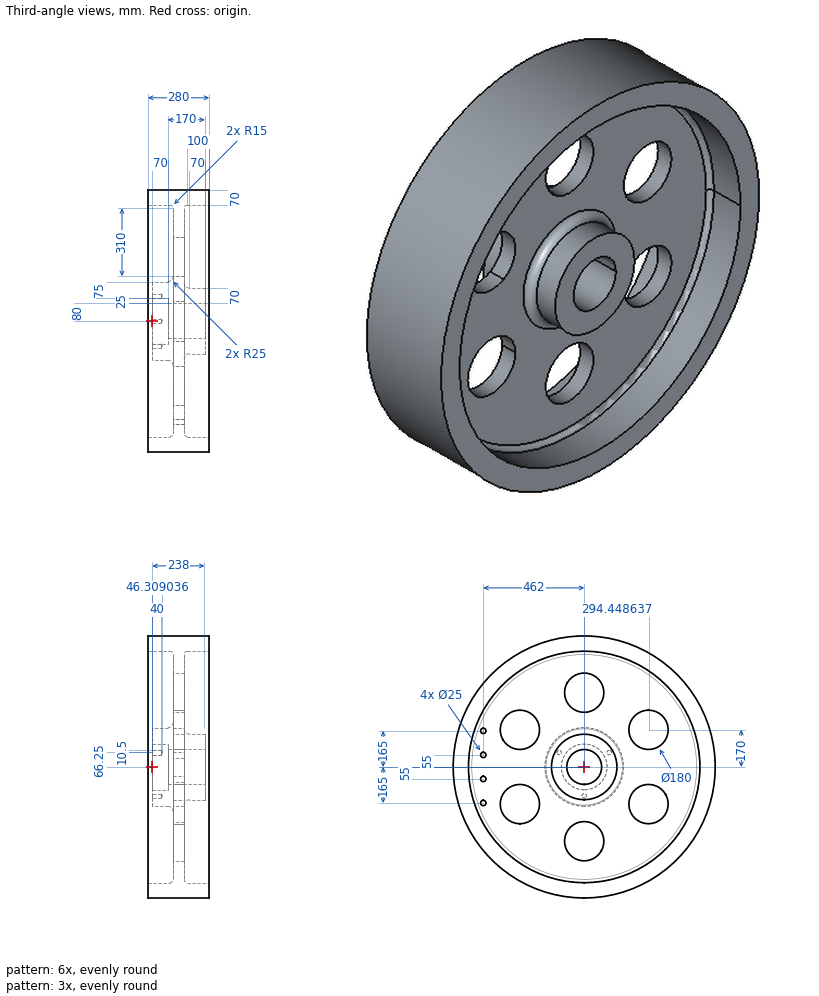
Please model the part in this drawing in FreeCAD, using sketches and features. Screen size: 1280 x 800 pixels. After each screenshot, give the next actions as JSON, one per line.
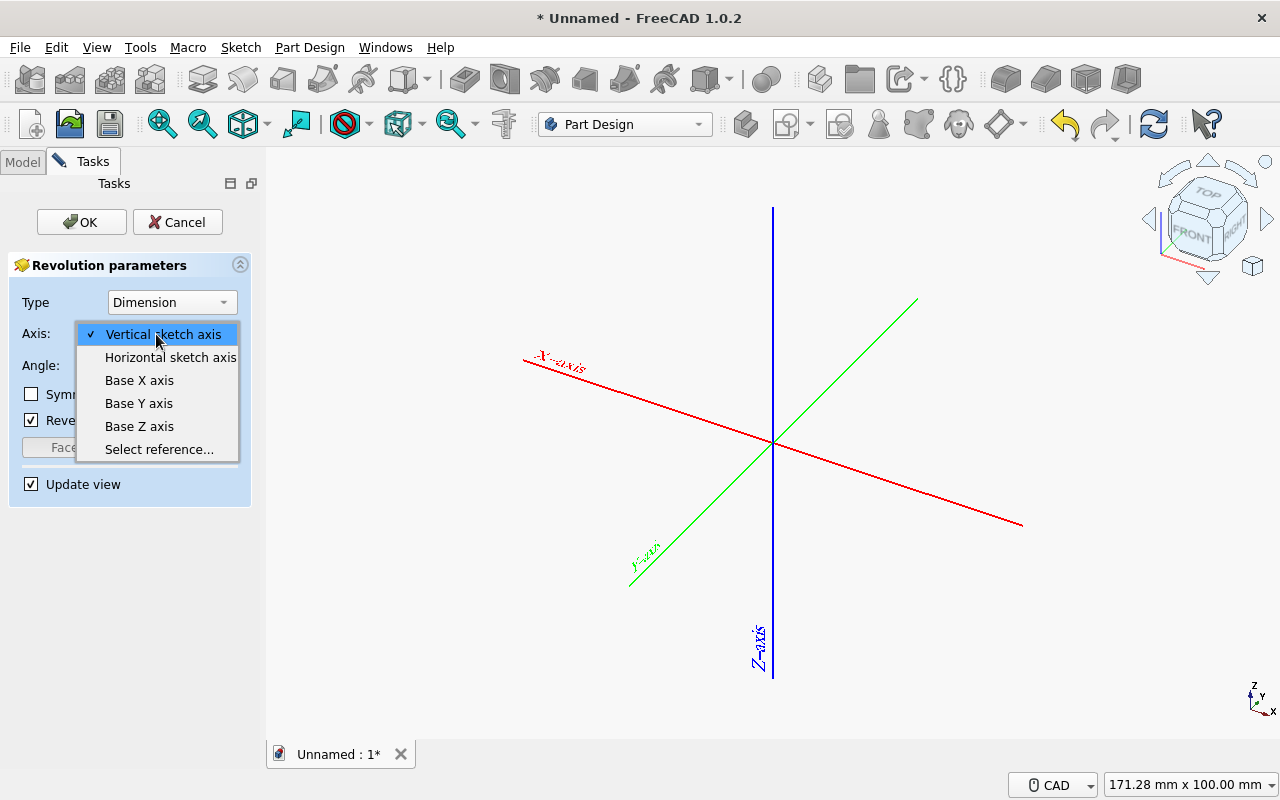
{"action": "left_click", "coordinate": [156, 358]}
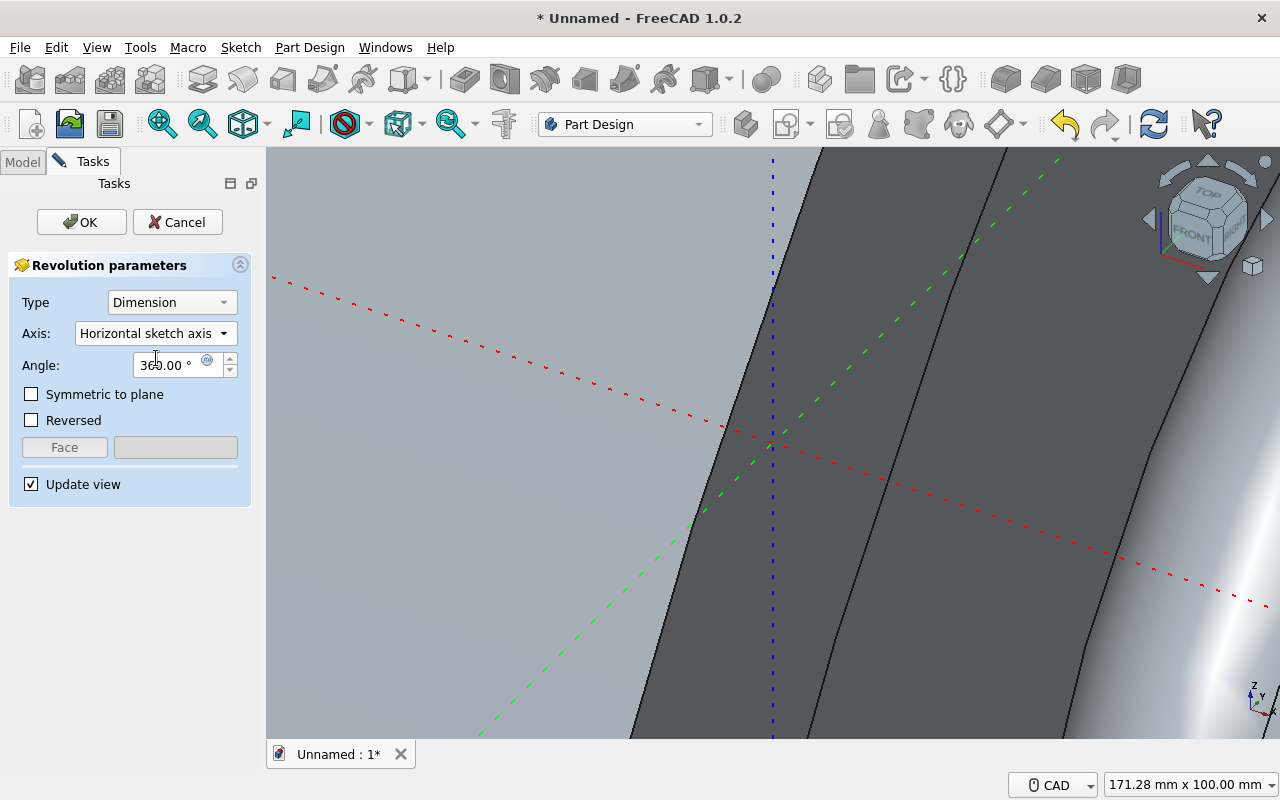
{"action": "left_click", "coordinate": [82, 222]}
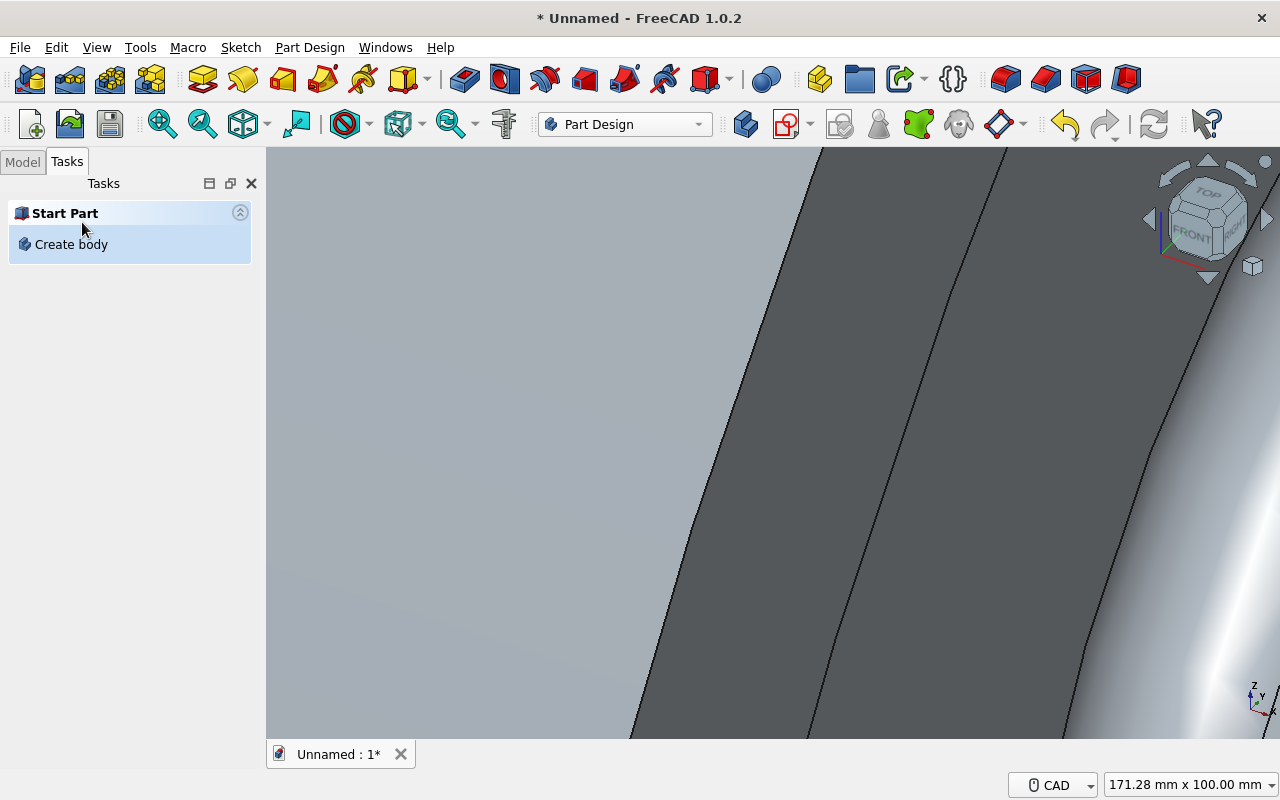
{"action": "left_click", "coordinate": [164, 124]}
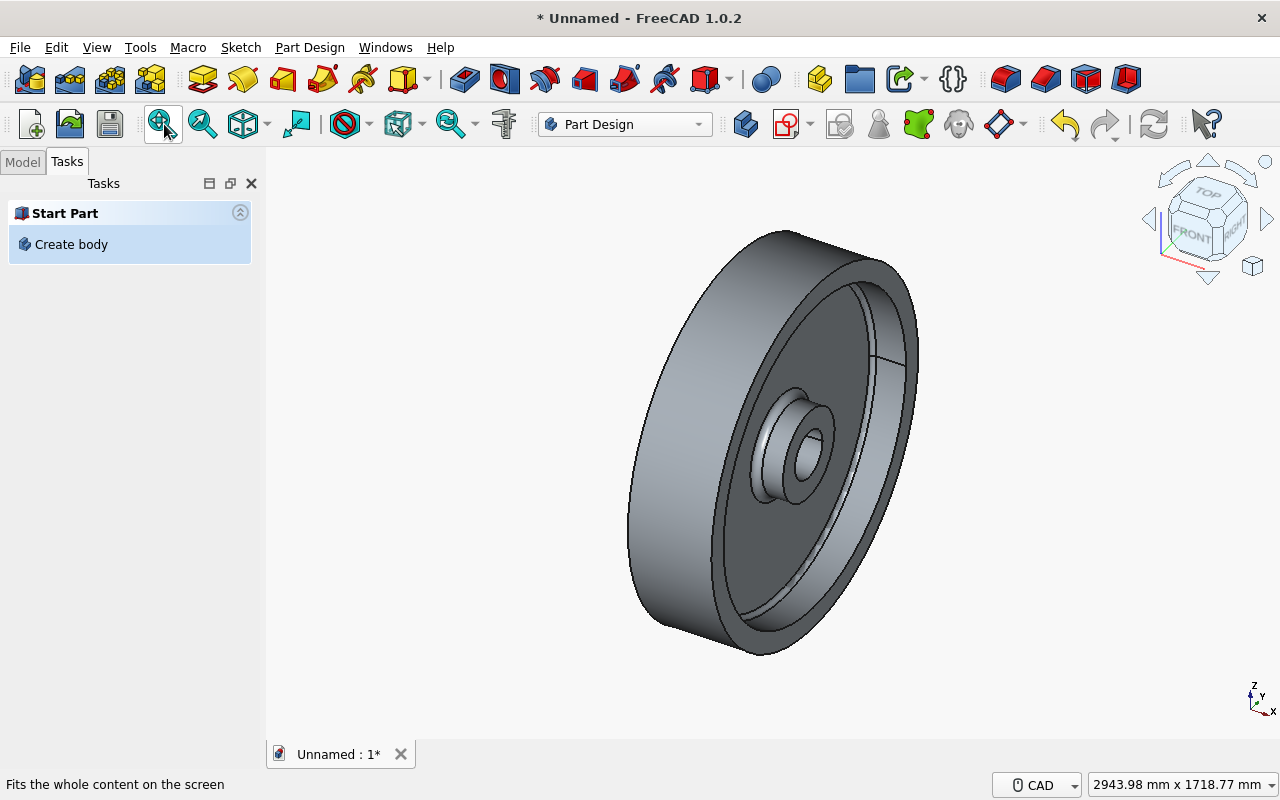
{"action": "key", "text": "6"}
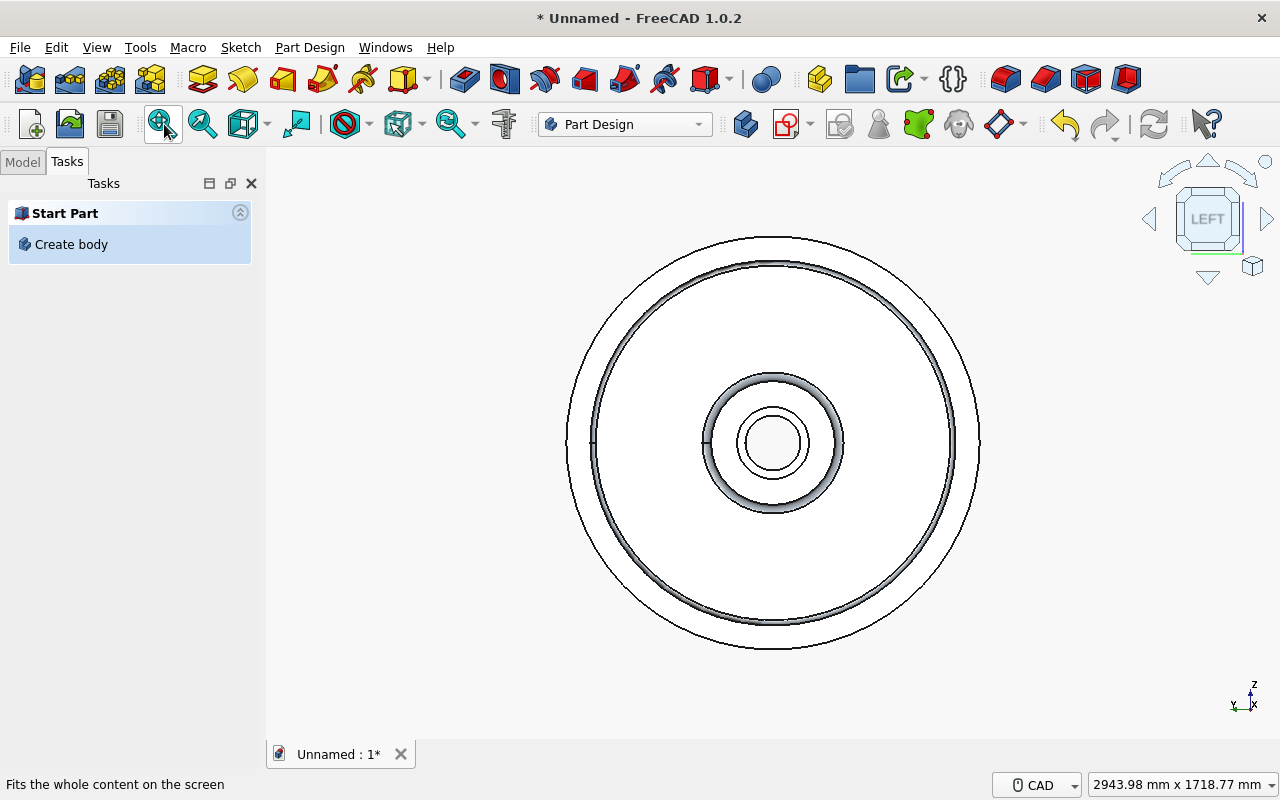
{"action": "left_click", "coordinate": [738, 407]}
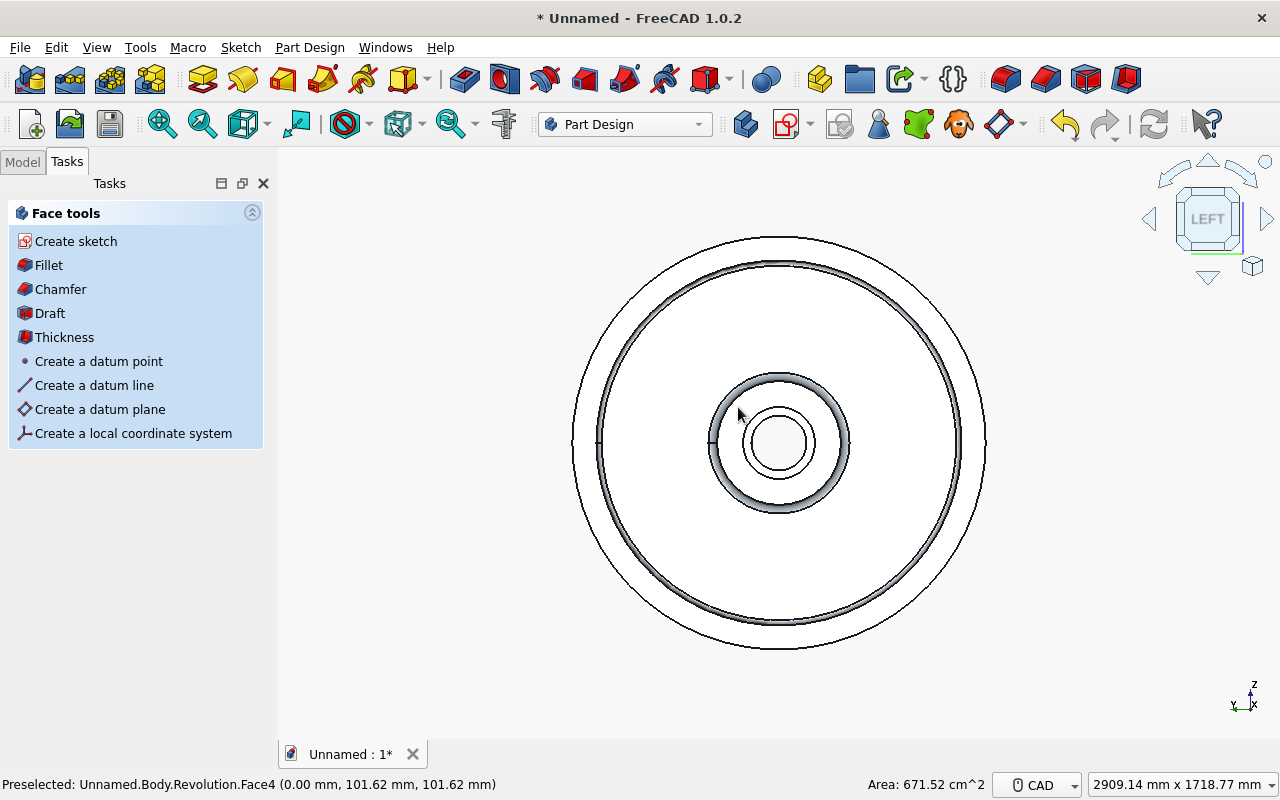
{"action": "left_click", "coordinate": [786, 124]}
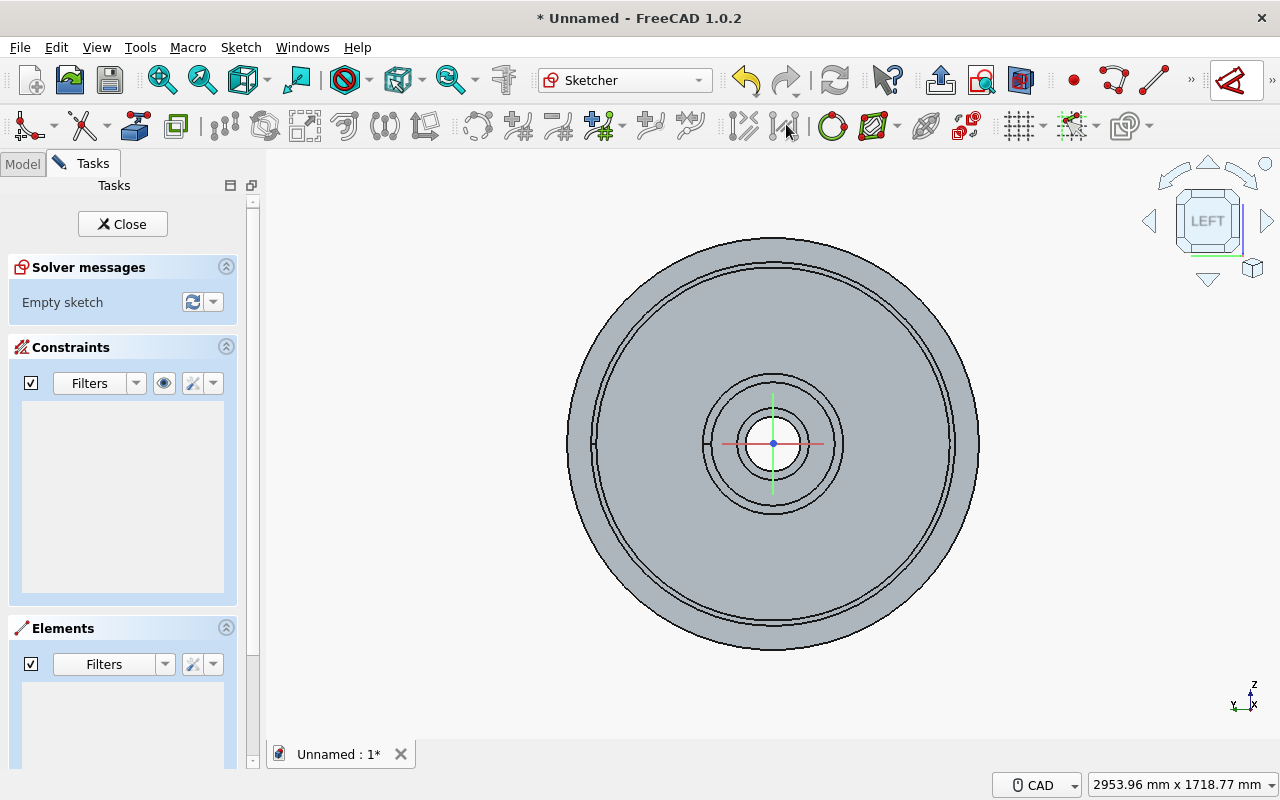
{"action": "scroll", "coordinate": [708, 385], "scroll_direction": "up", "scroll_amount": 7}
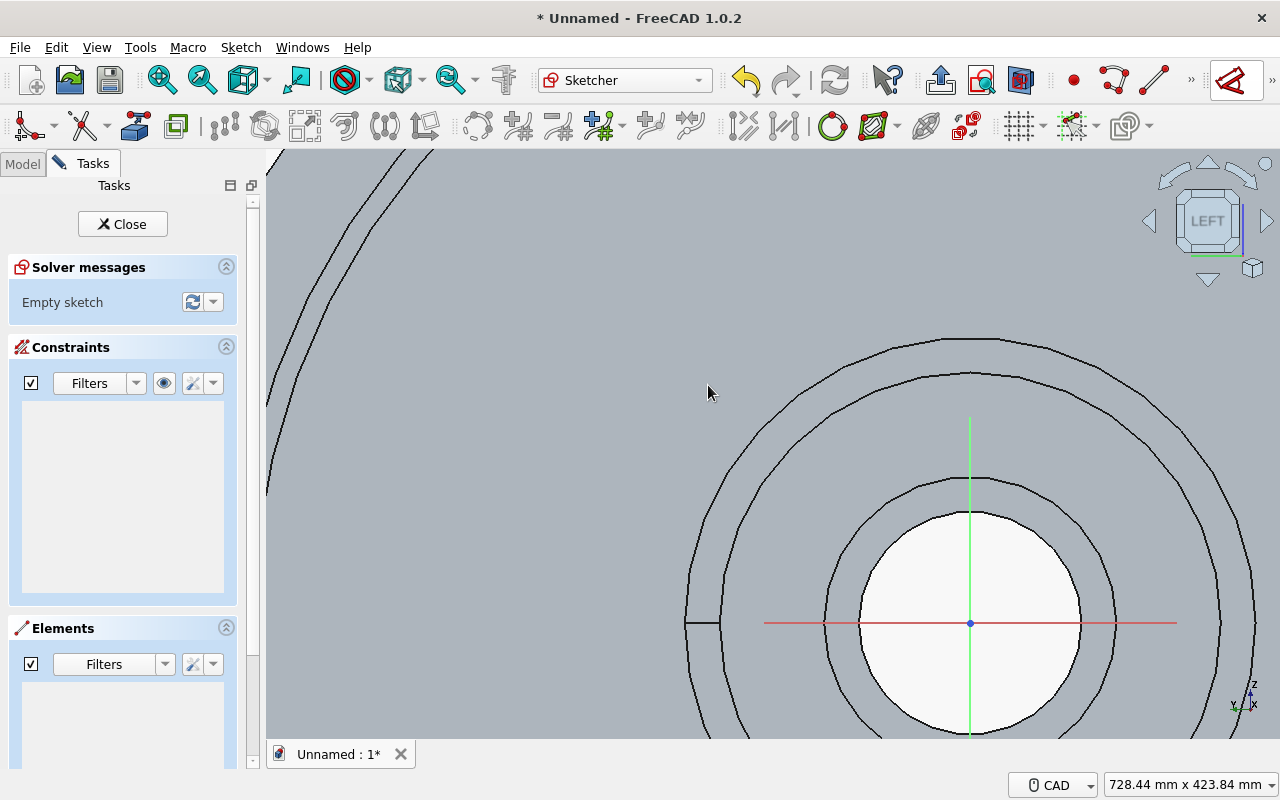
{"action": "key", "text": "g c"}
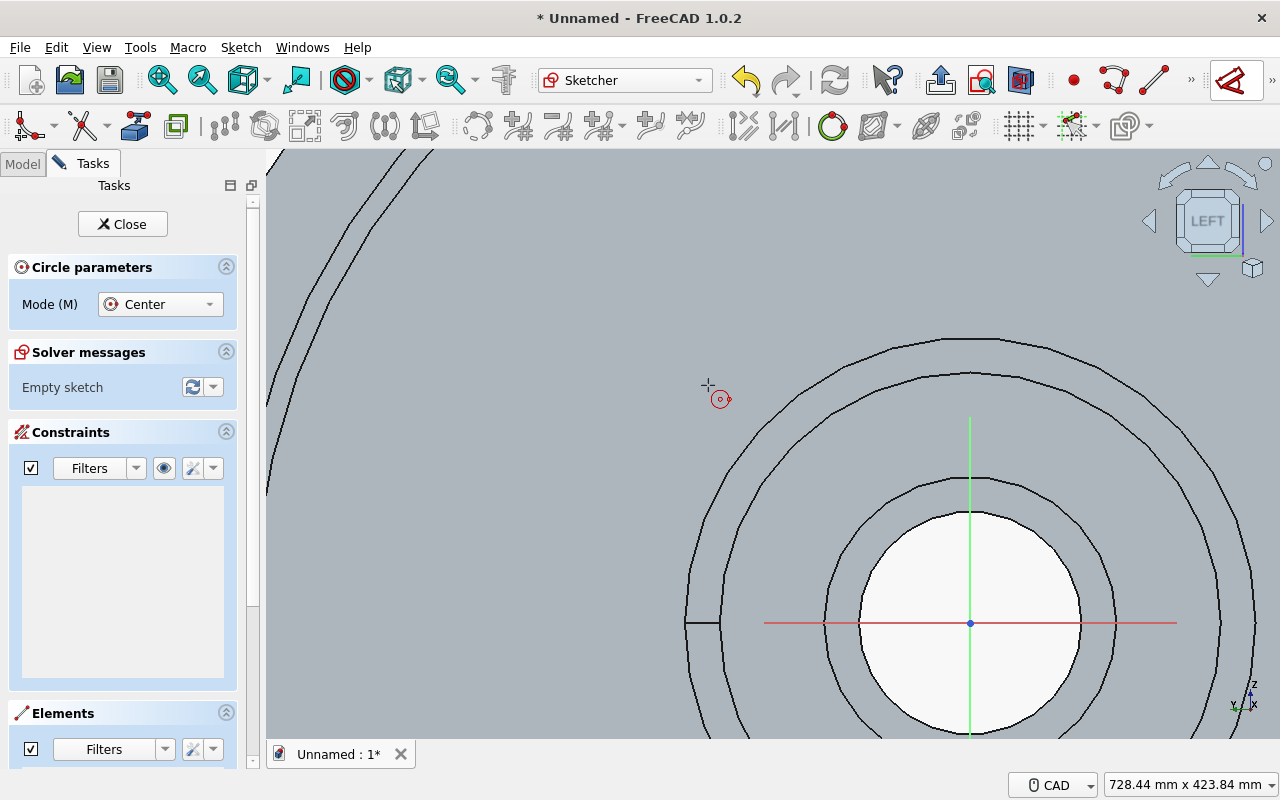
{"action": "left_click", "coordinate": [560, 386]}
{"action": "left_click", "coordinate": [649, 298]}
{"action": "key", "text": "Escape"}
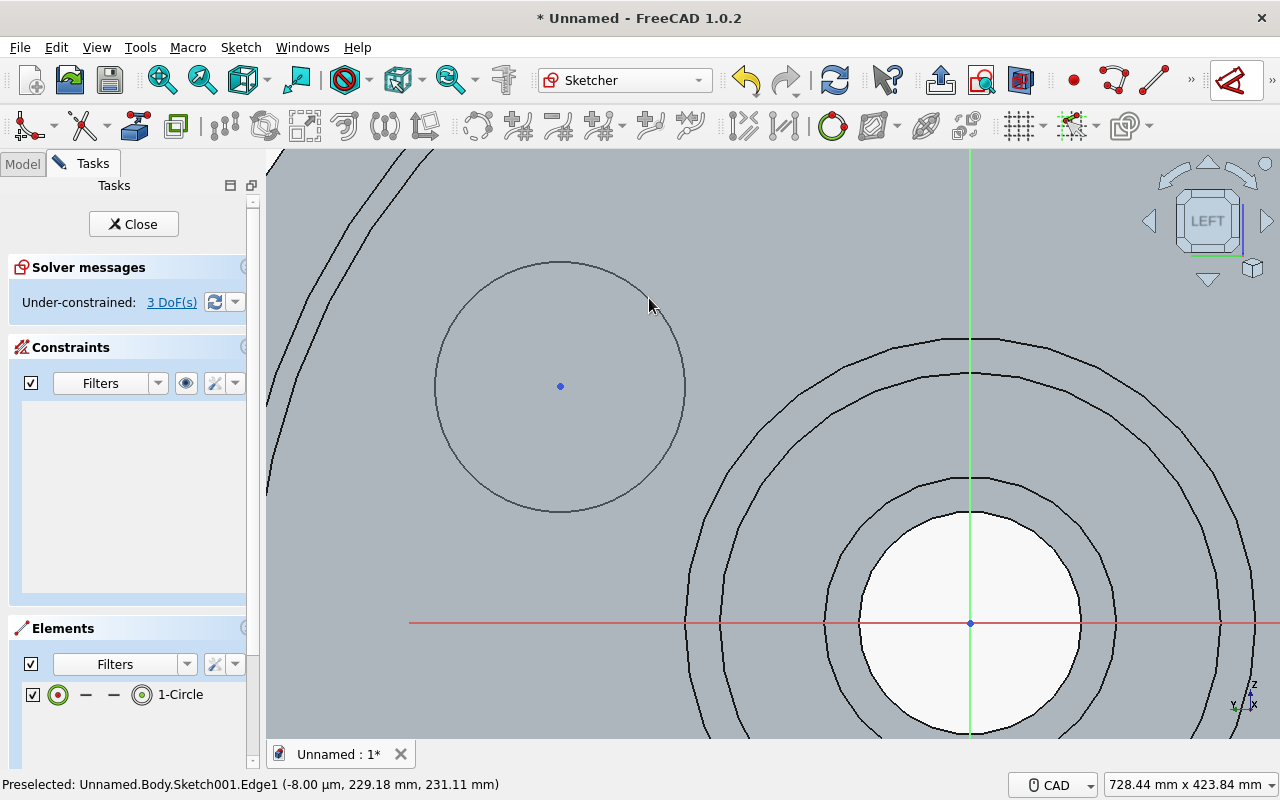
{"action": "left_click", "coordinate": [648, 298]}